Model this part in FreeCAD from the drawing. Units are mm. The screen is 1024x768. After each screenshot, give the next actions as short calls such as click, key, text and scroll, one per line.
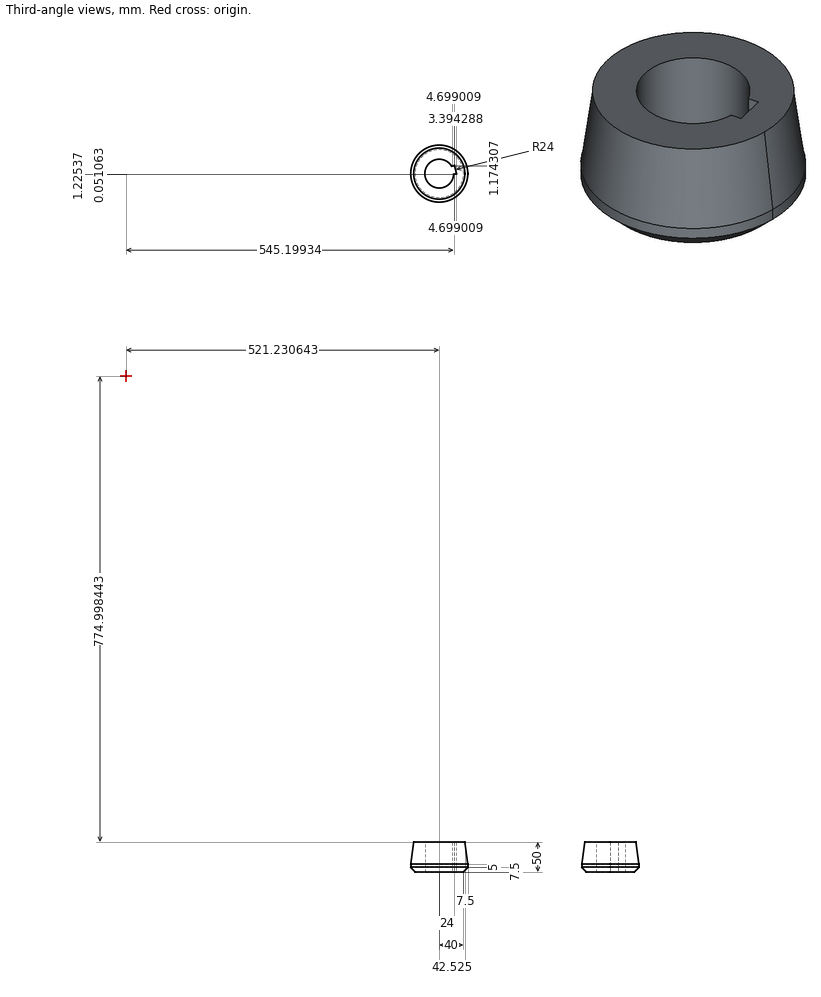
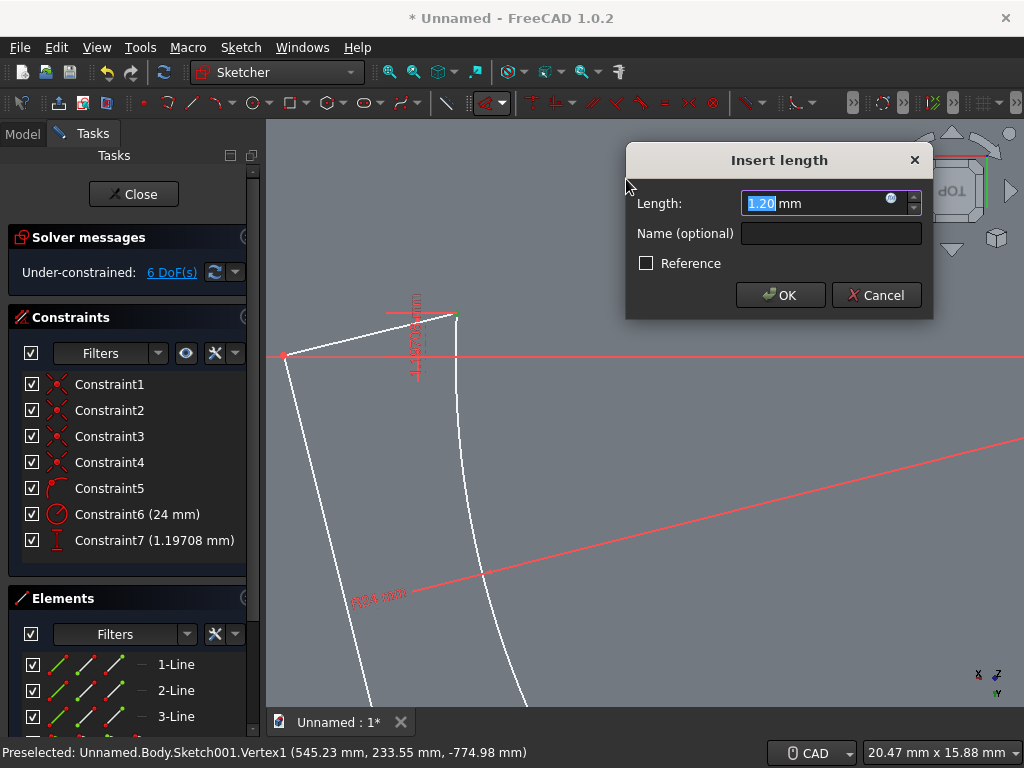
text(1.22537)
key(Return)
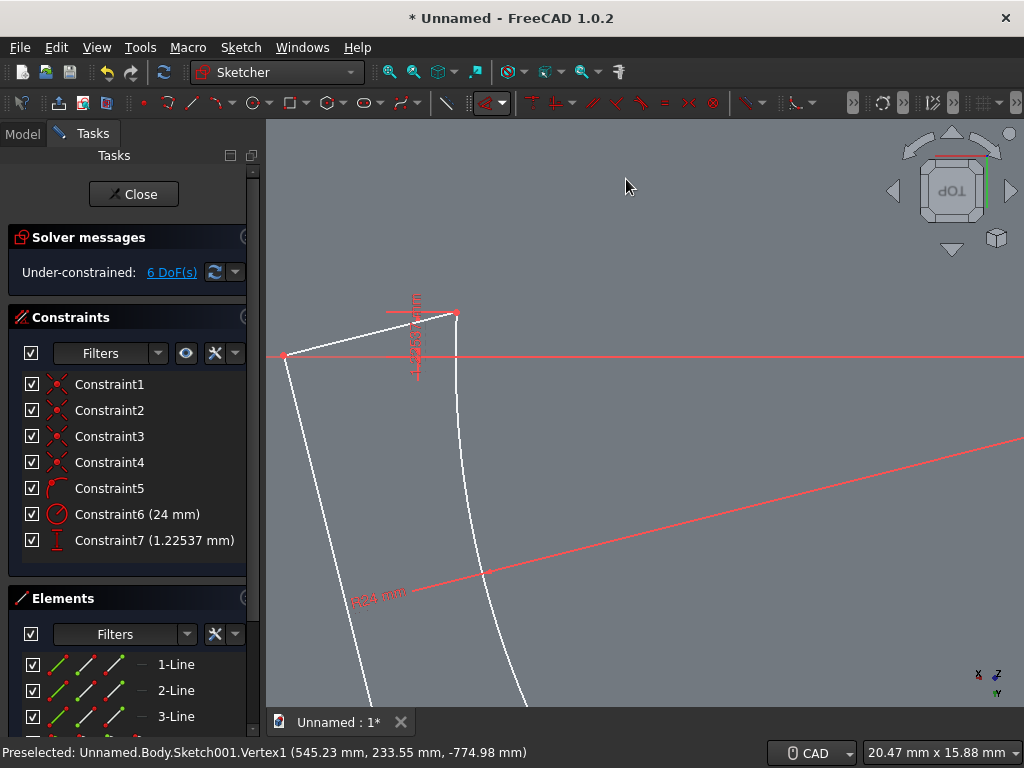
scroll(859, 147, down, 2)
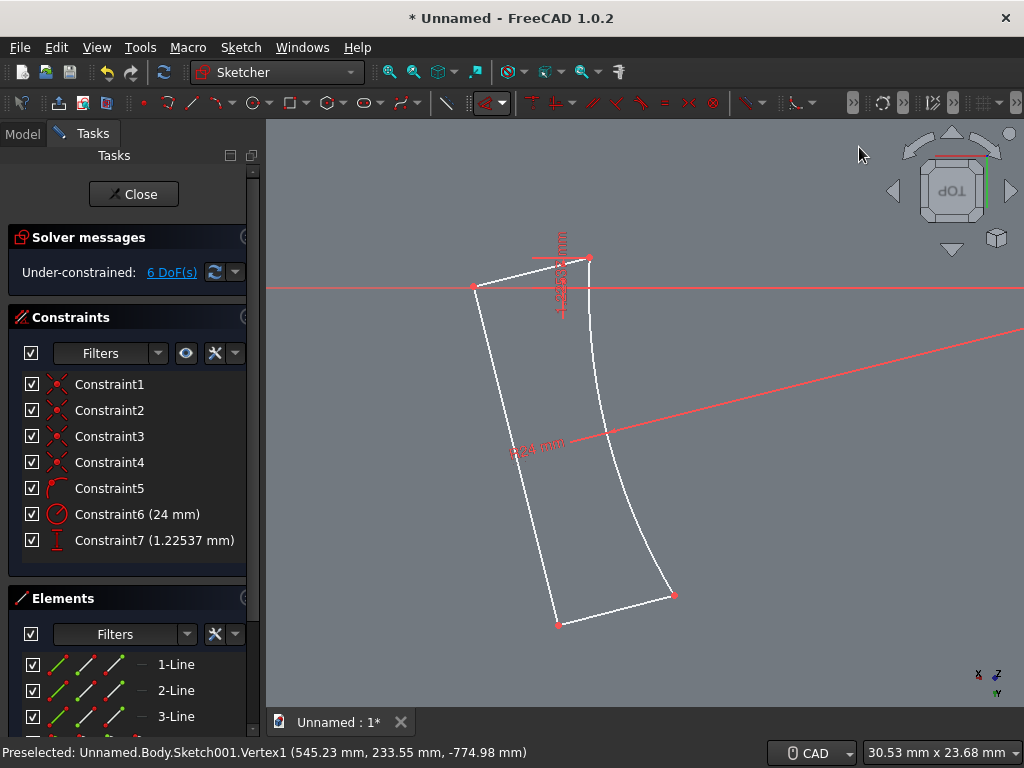
scroll(474, 287, up, 18)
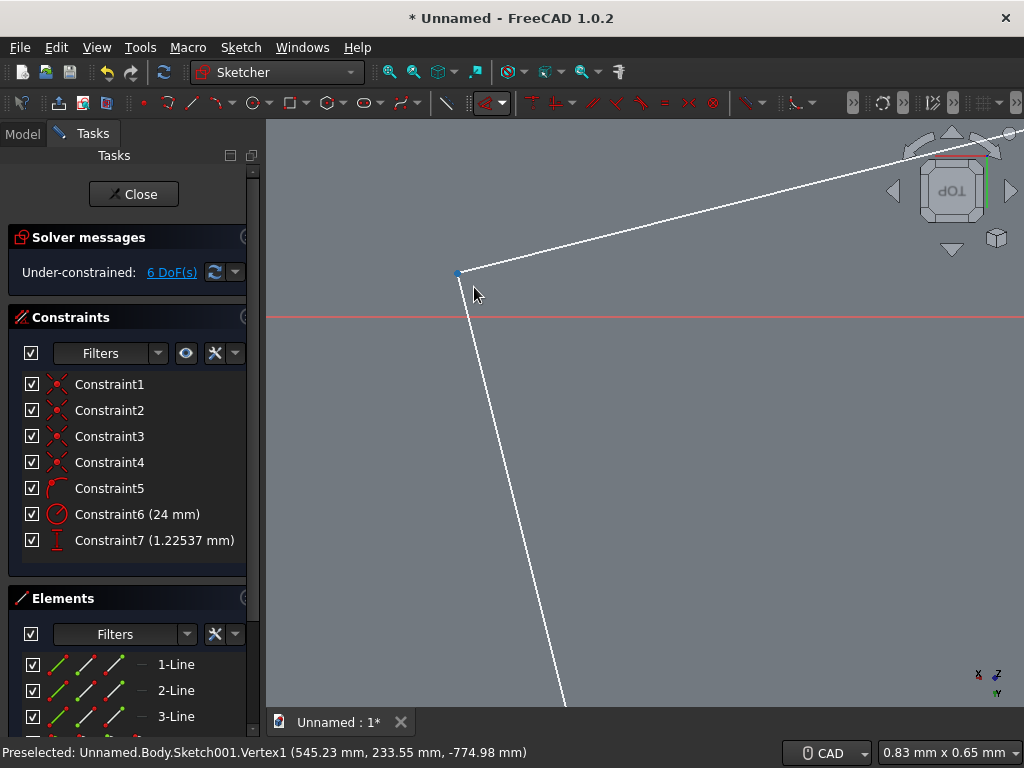
click(457, 273)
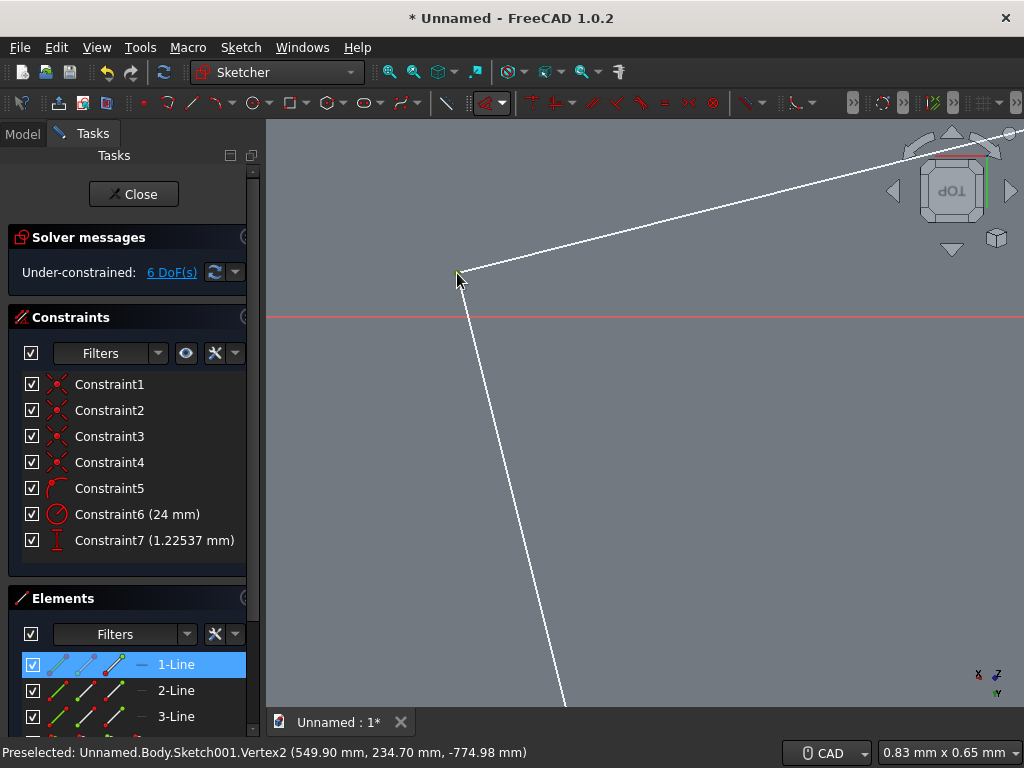
key(i)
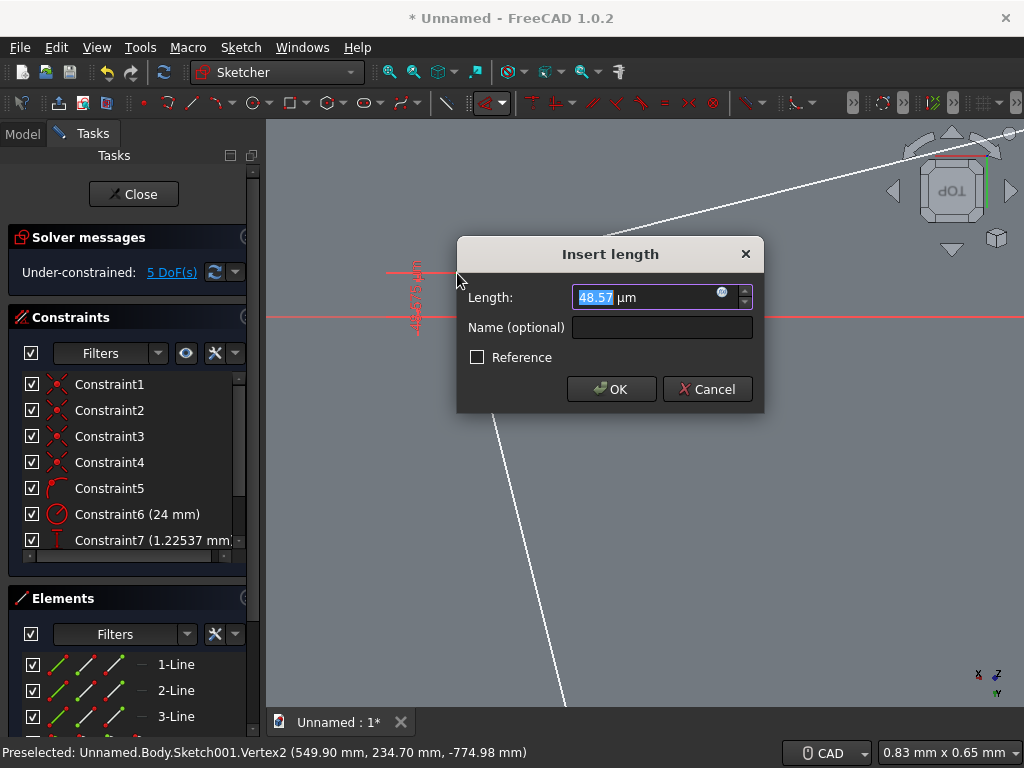
key(ctrl+a)
text(0.051063 mm)
key(Return)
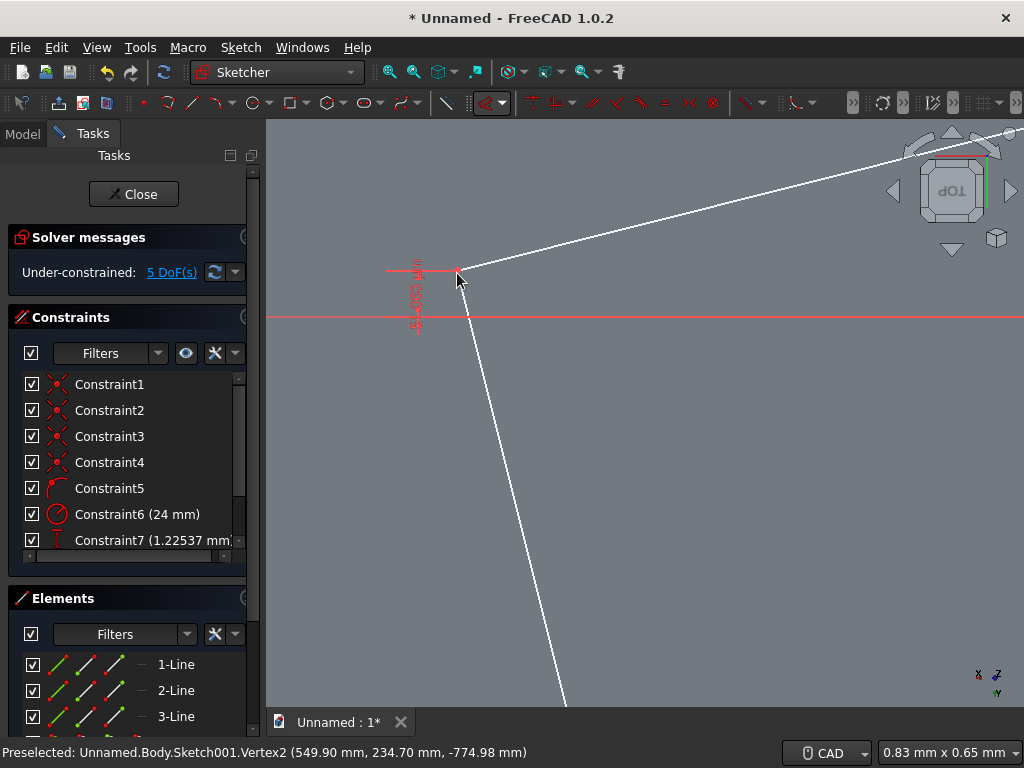
scroll(454, 223, down, 17)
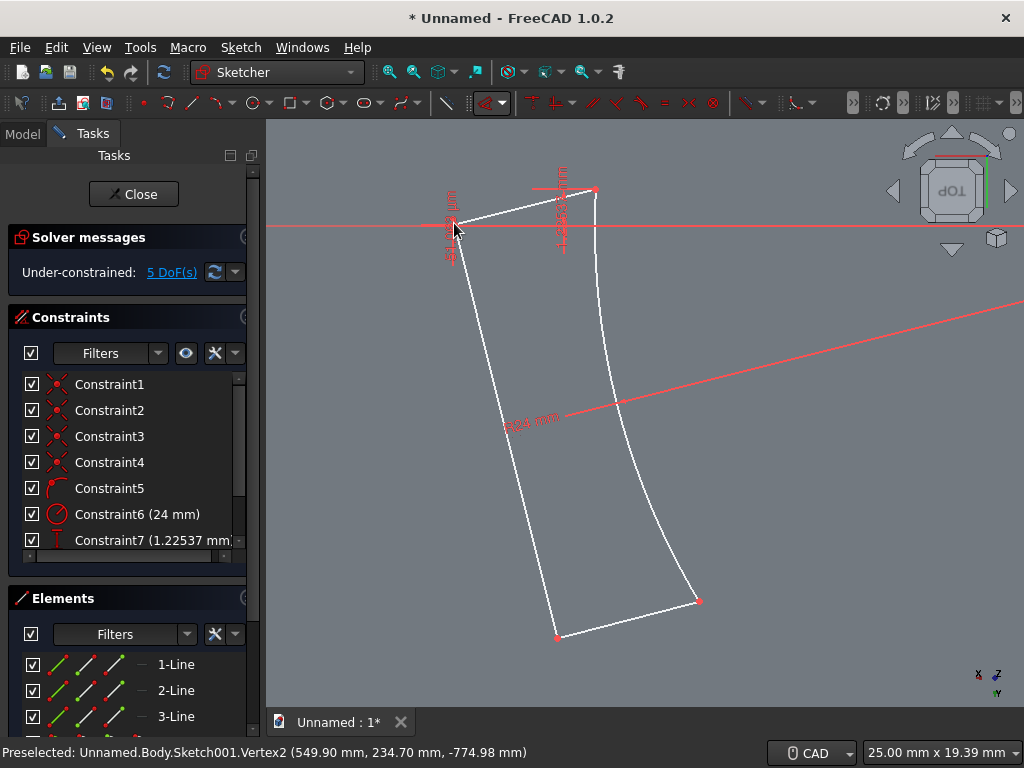
click(553, 200)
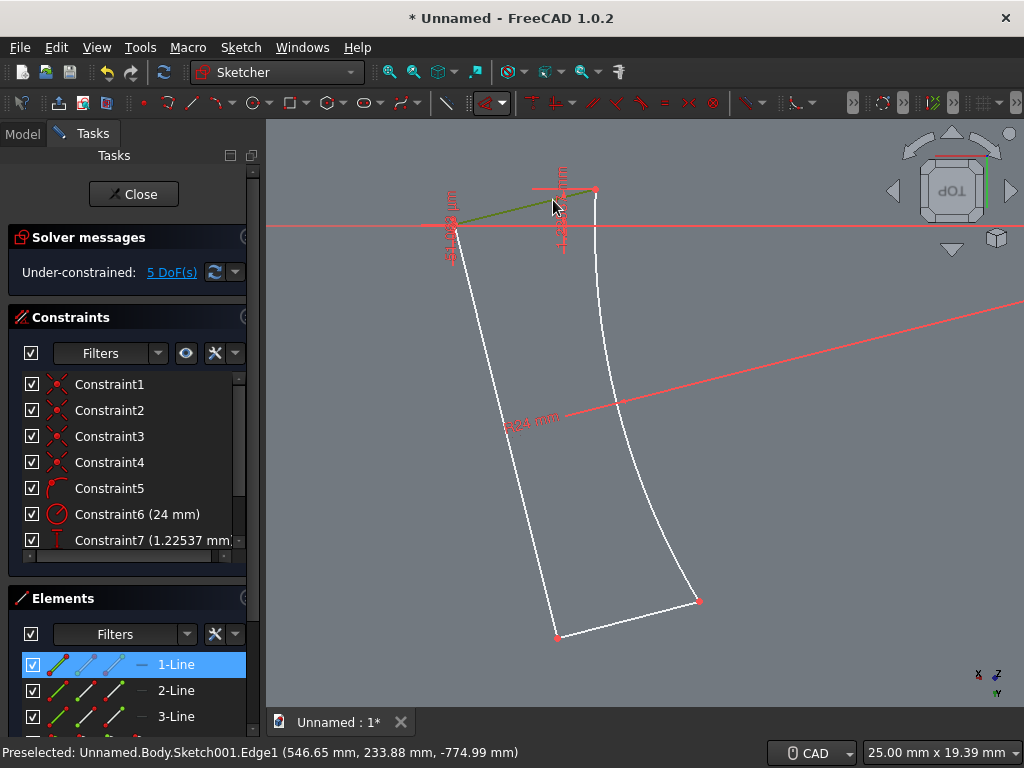
click(504, 104)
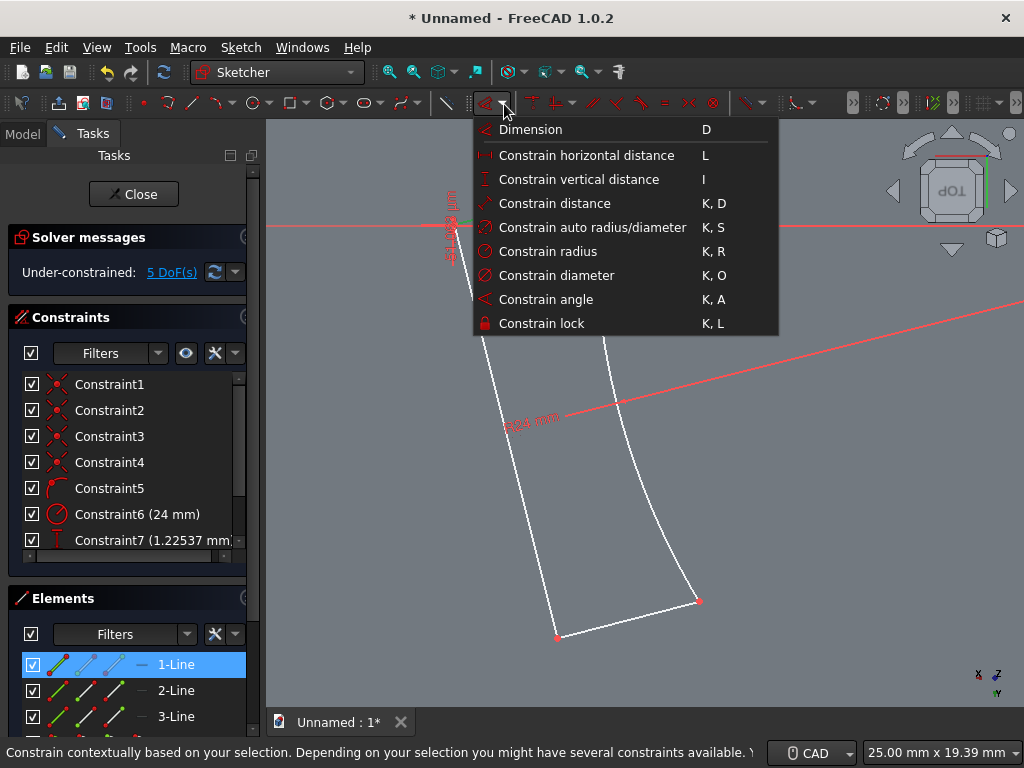
click(626, 155)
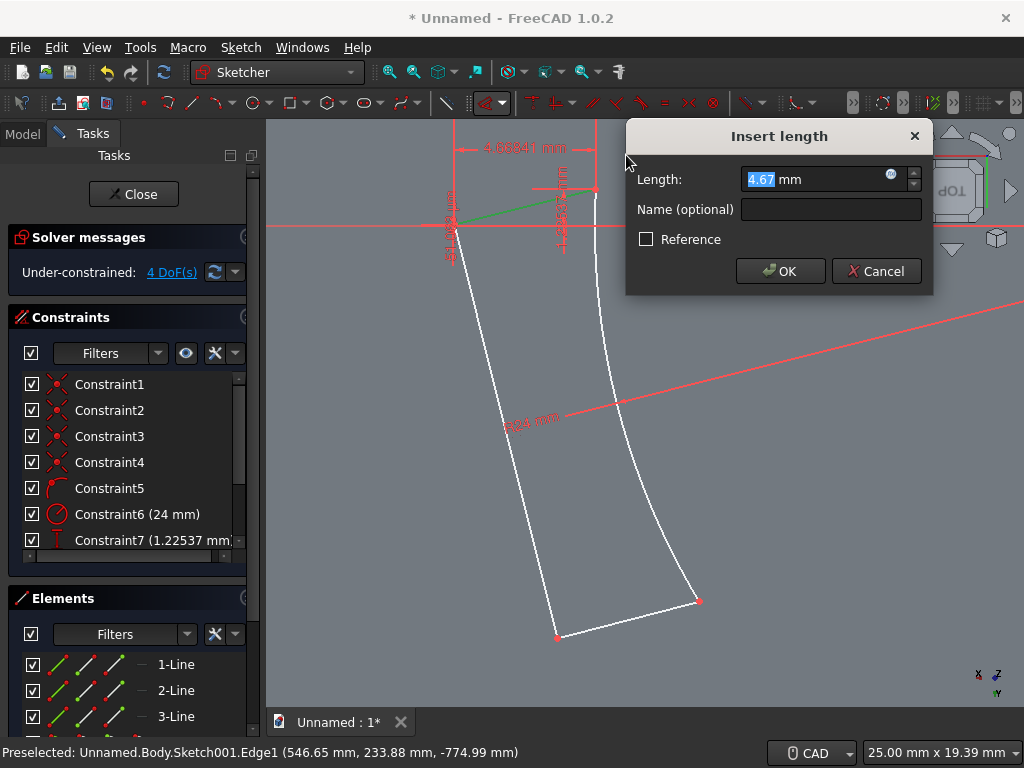
text(4.699009)
key(Return)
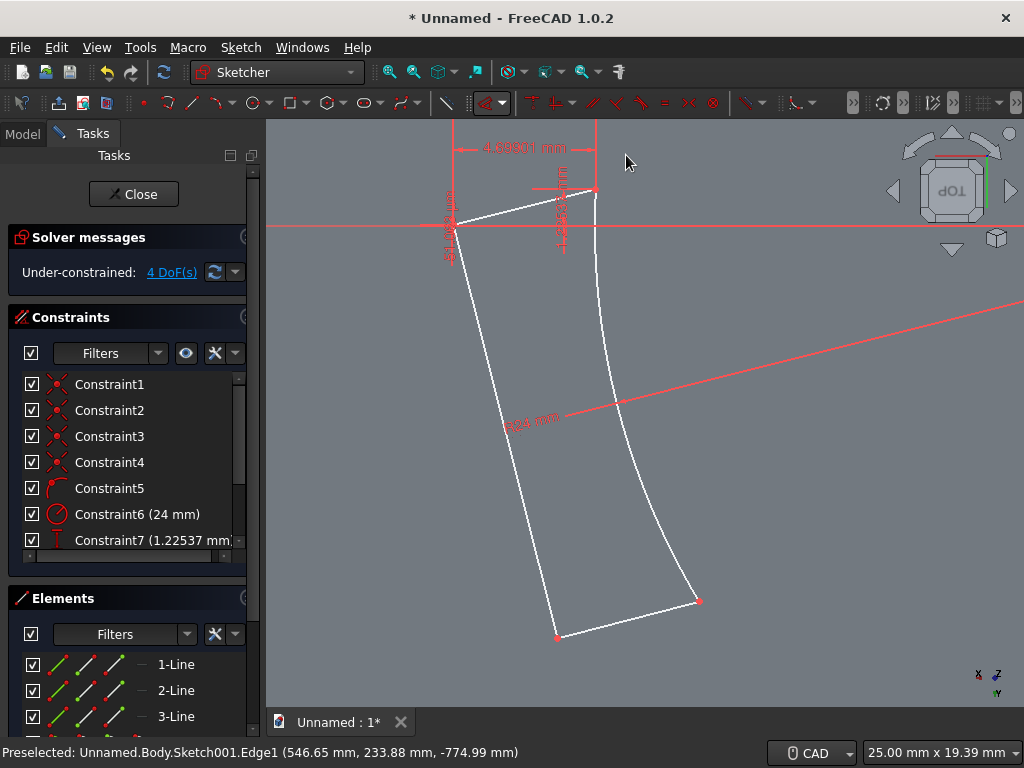
click(485, 349)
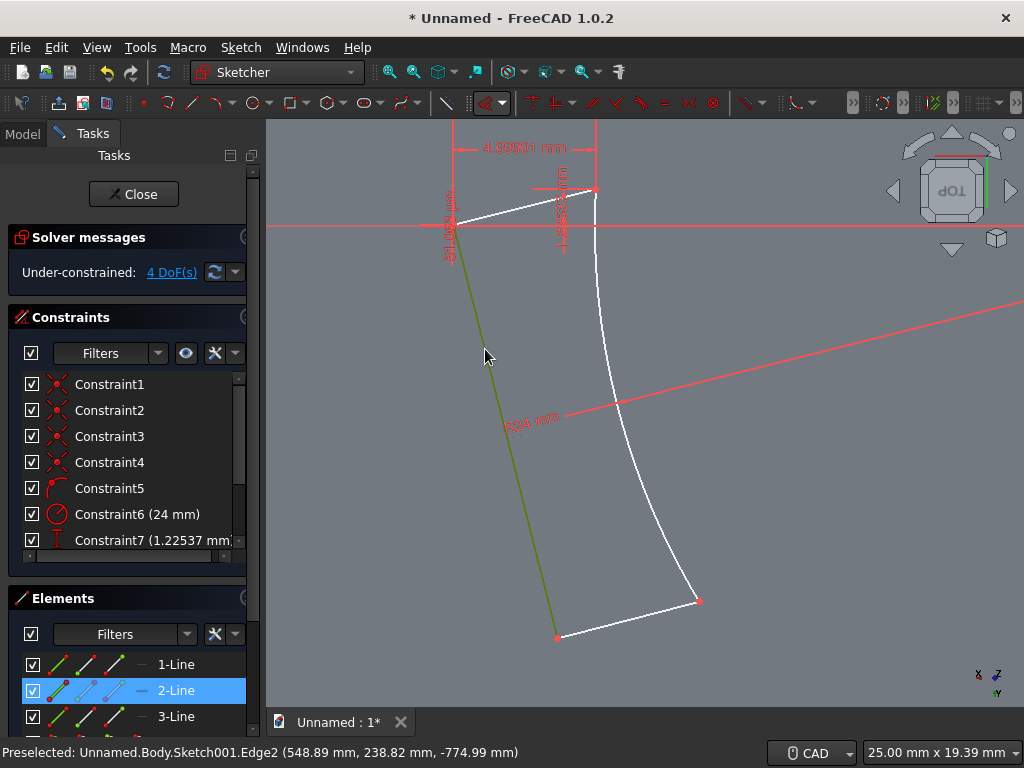
key(l)